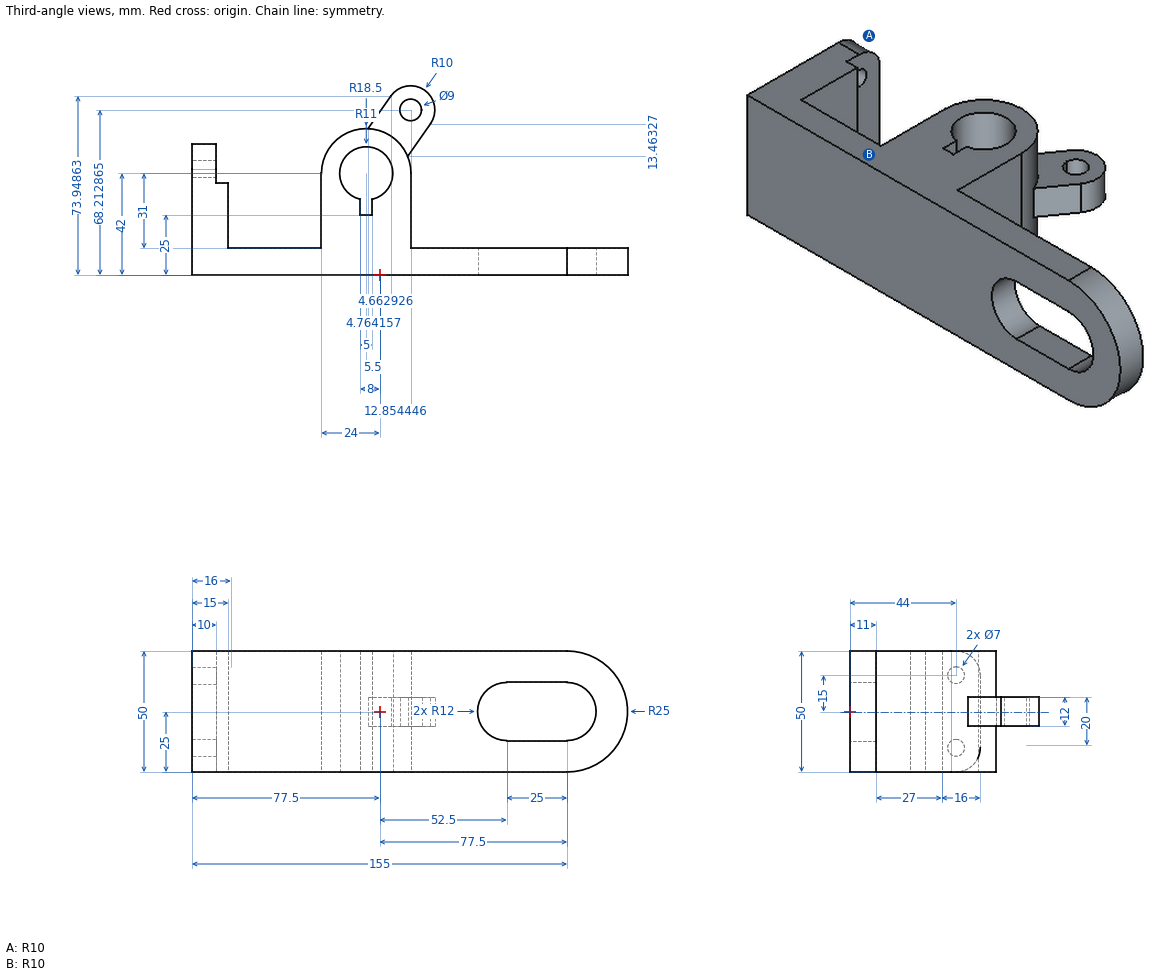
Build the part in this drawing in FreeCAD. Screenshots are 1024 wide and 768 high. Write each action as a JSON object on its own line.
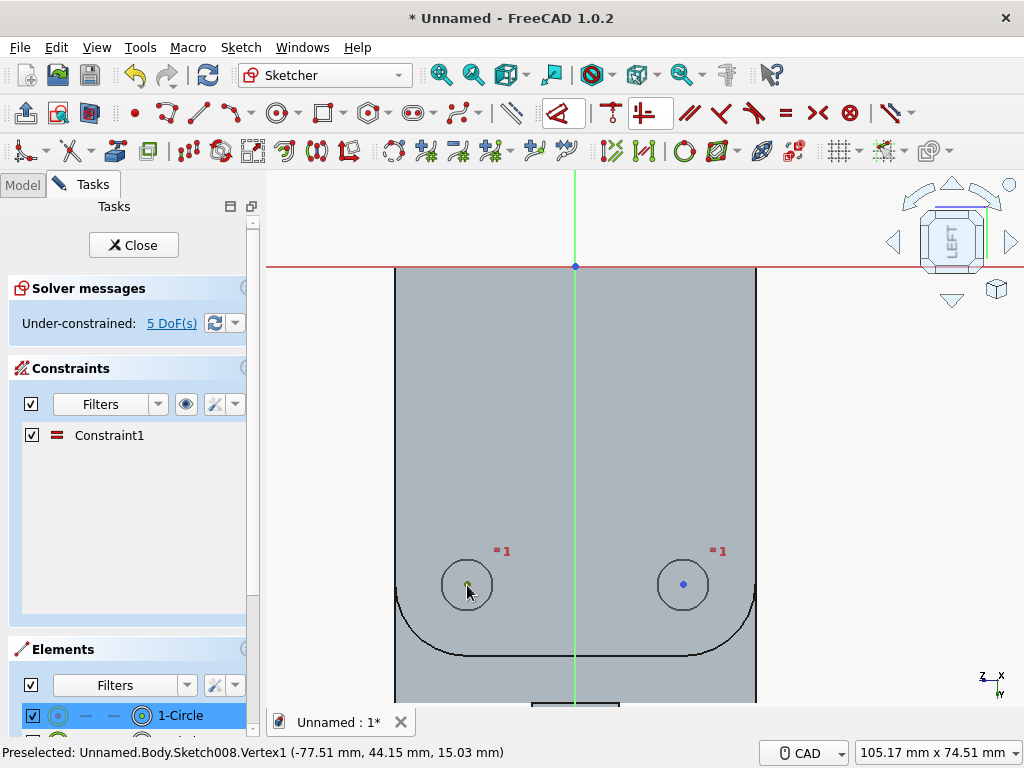
{"action": "left_click", "coordinate": [683, 585]}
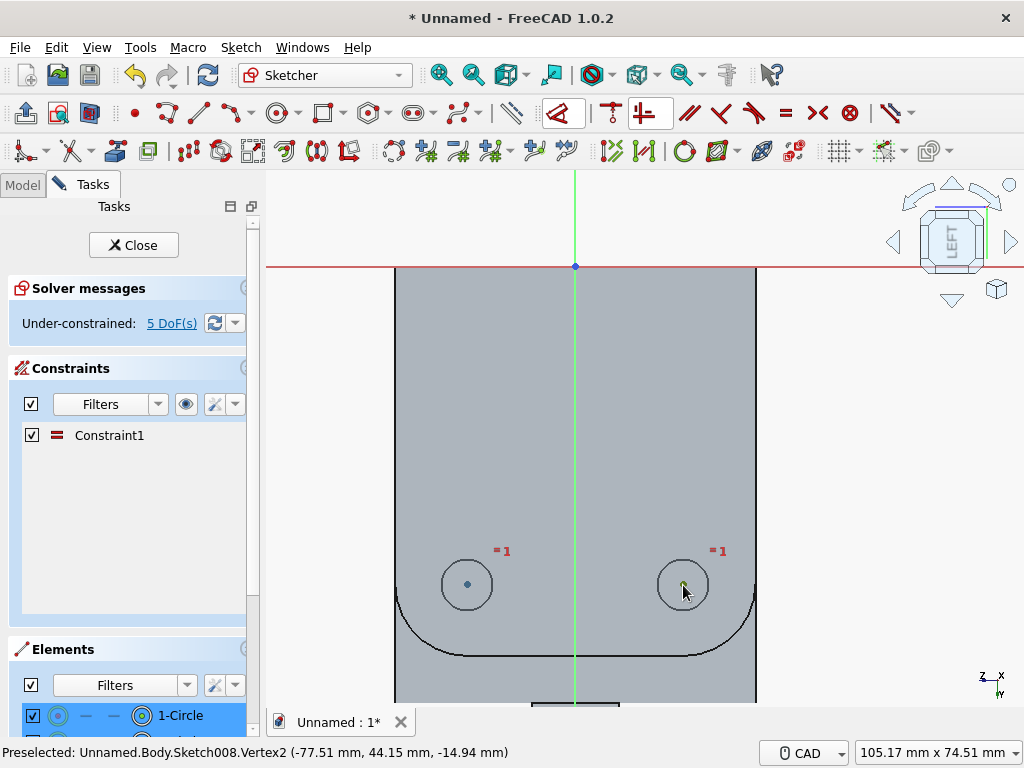
{"action": "left_click", "coordinate": [575, 645]}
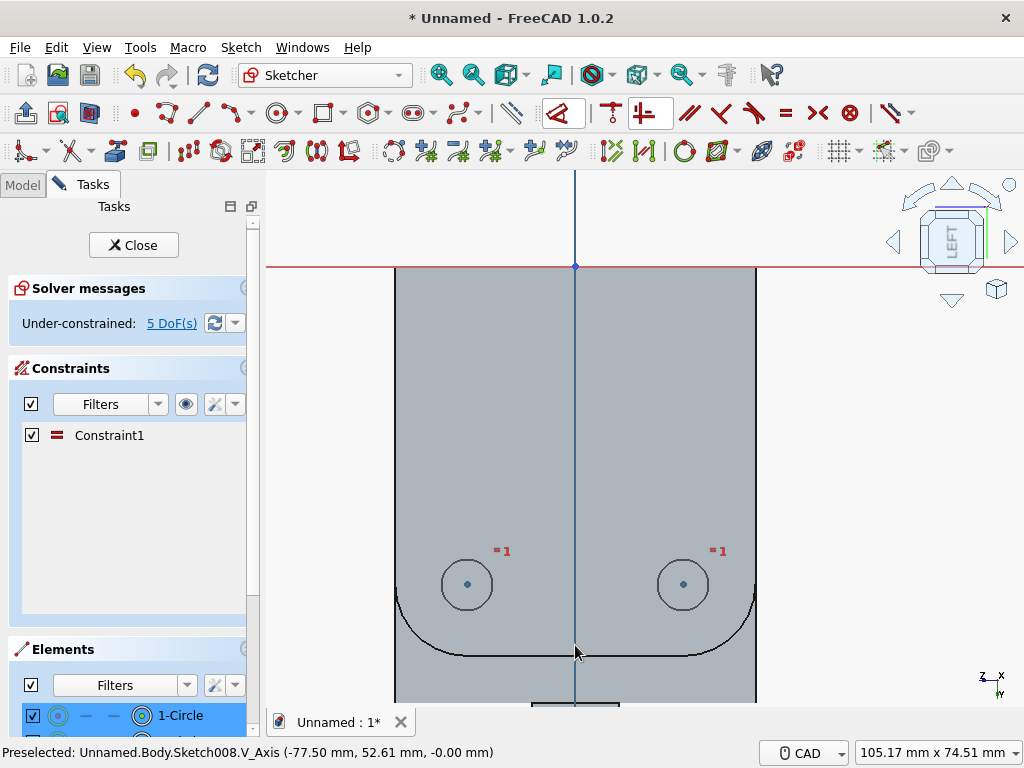
{"action": "left_click", "coordinate": [818, 114]}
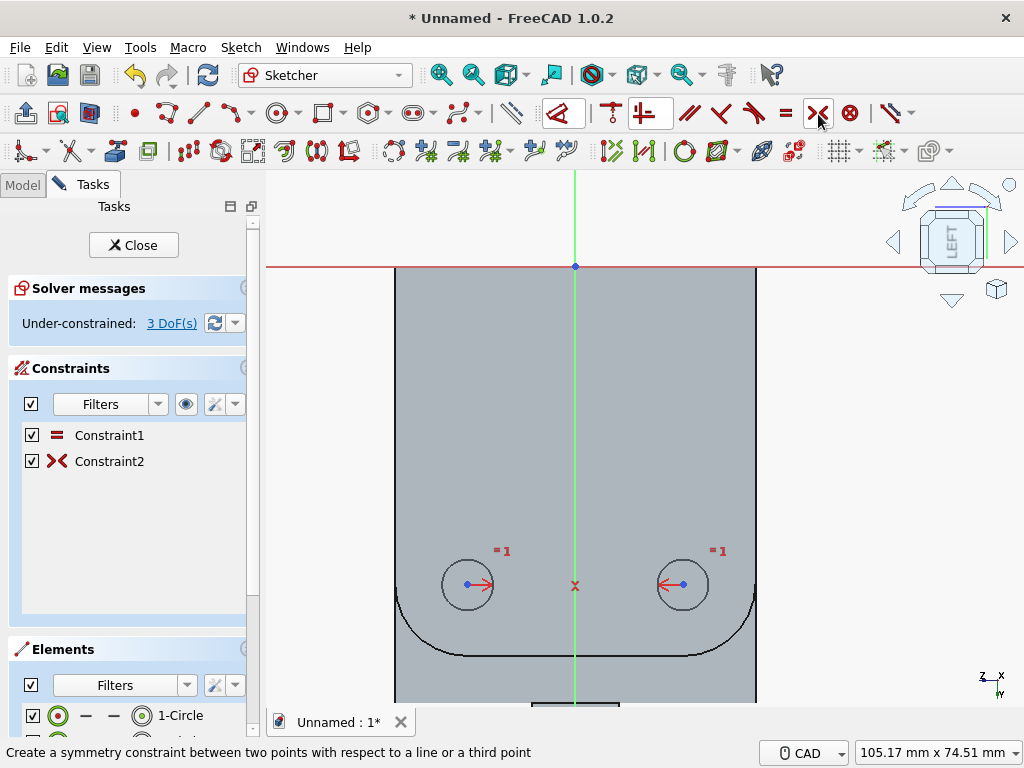
{"action": "left_click", "coordinate": [486, 567]}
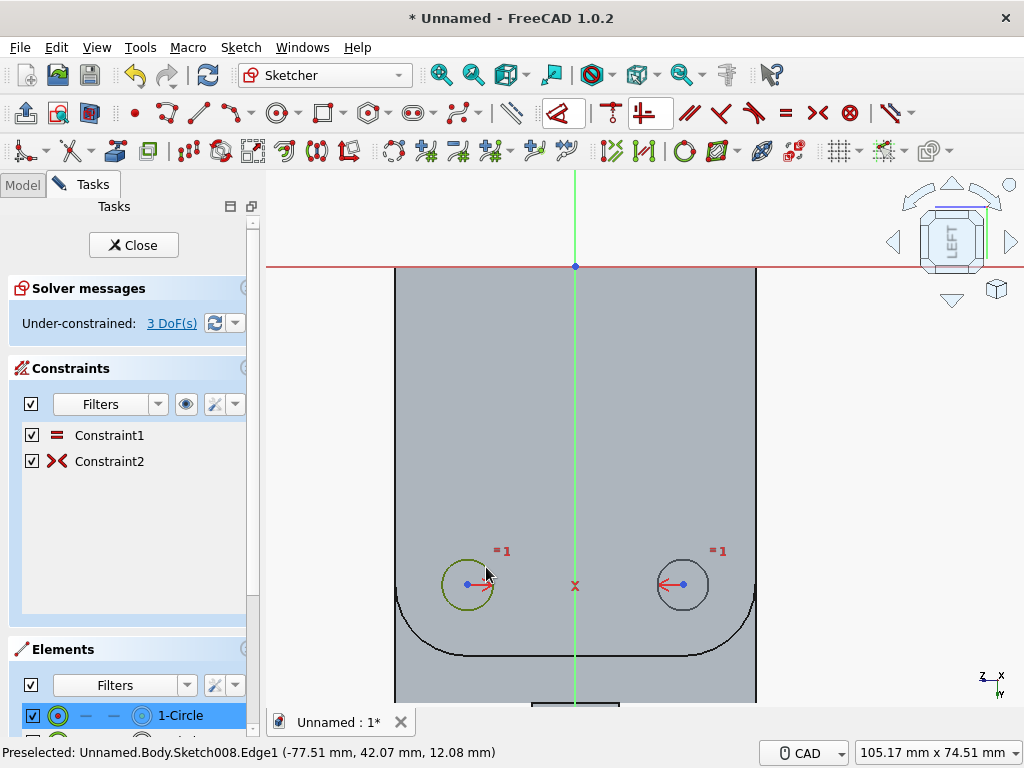
{"action": "key", "text": "k o"}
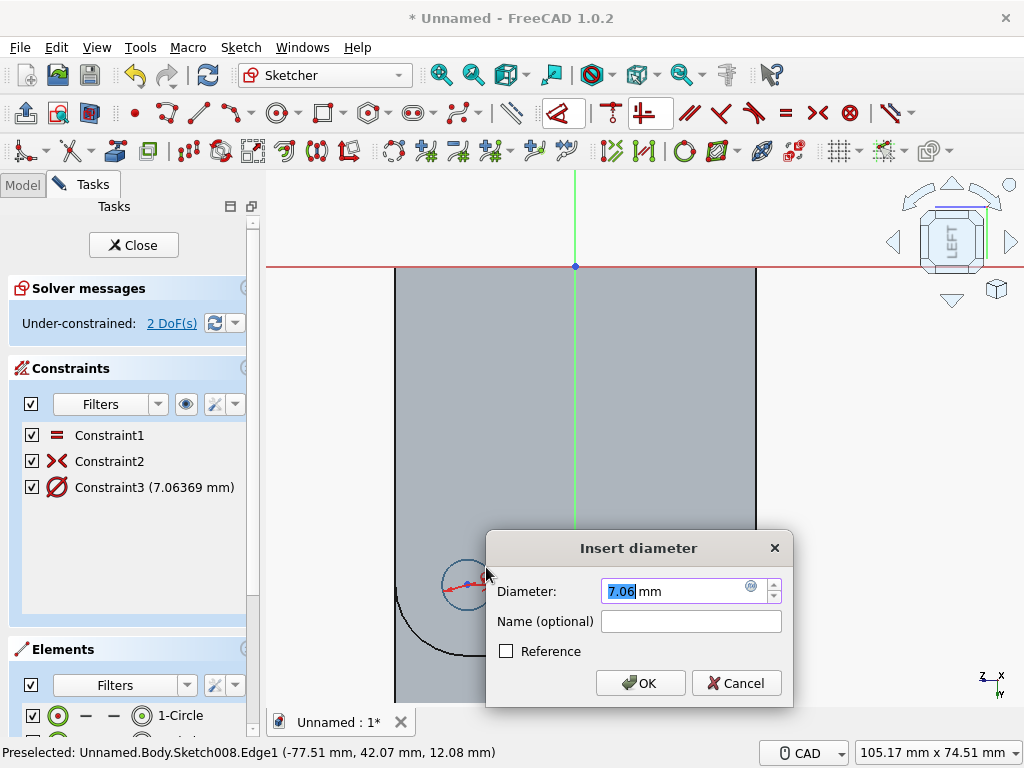
{"action": "type", "text": "7"}
{"action": "key", "text": "Return"}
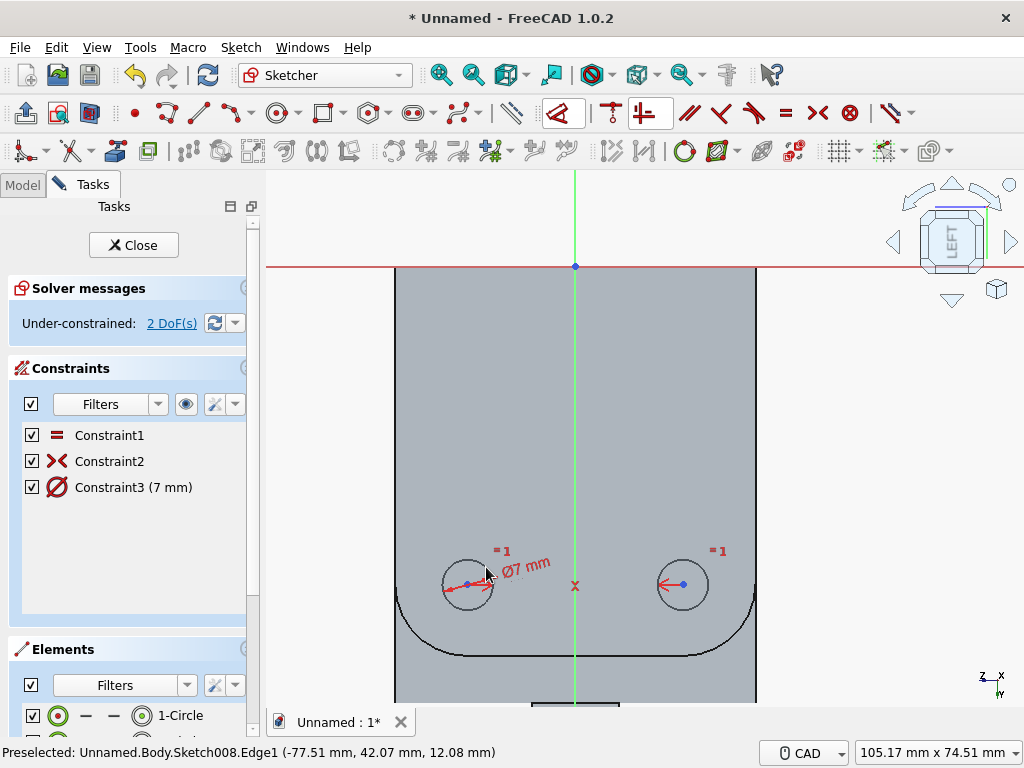
{"action": "left_click", "coordinate": [468, 585]}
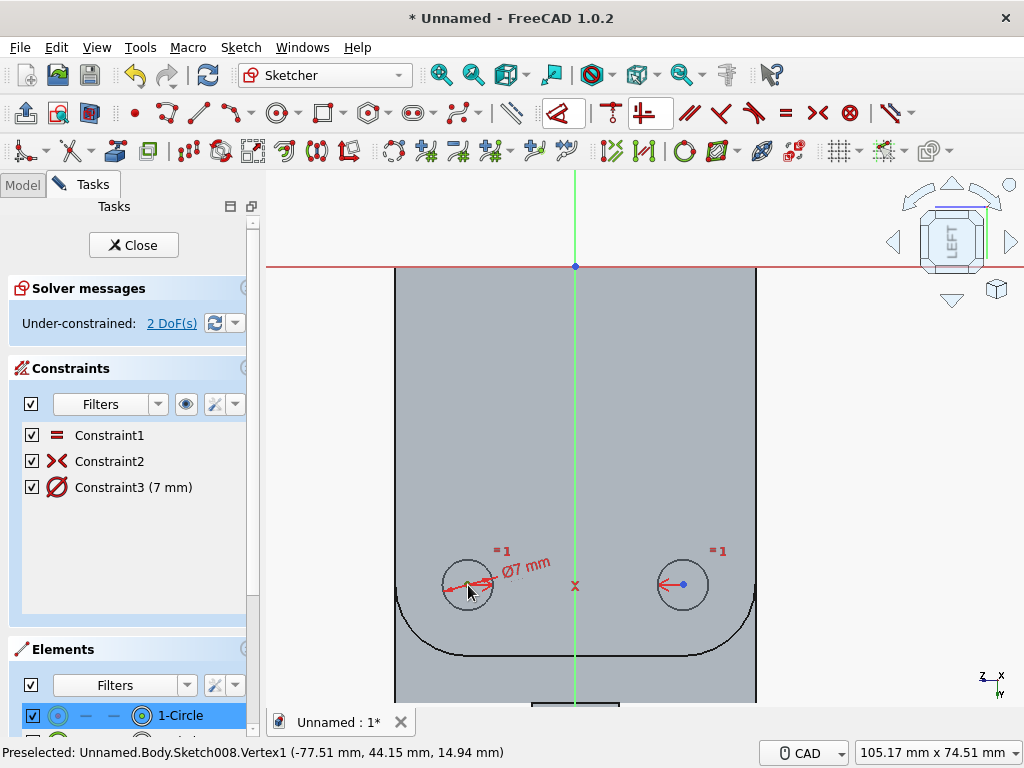
{"action": "left_click", "coordinate": [580, 114]}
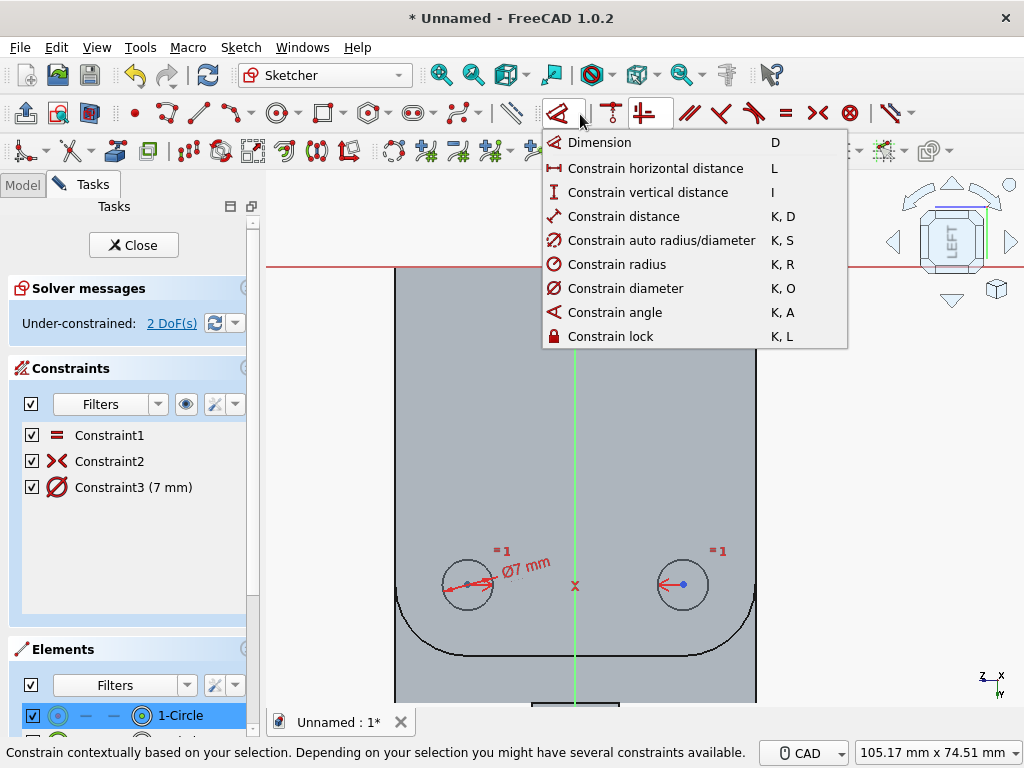
{"action": "left_click", "coordinate": [695, 168]}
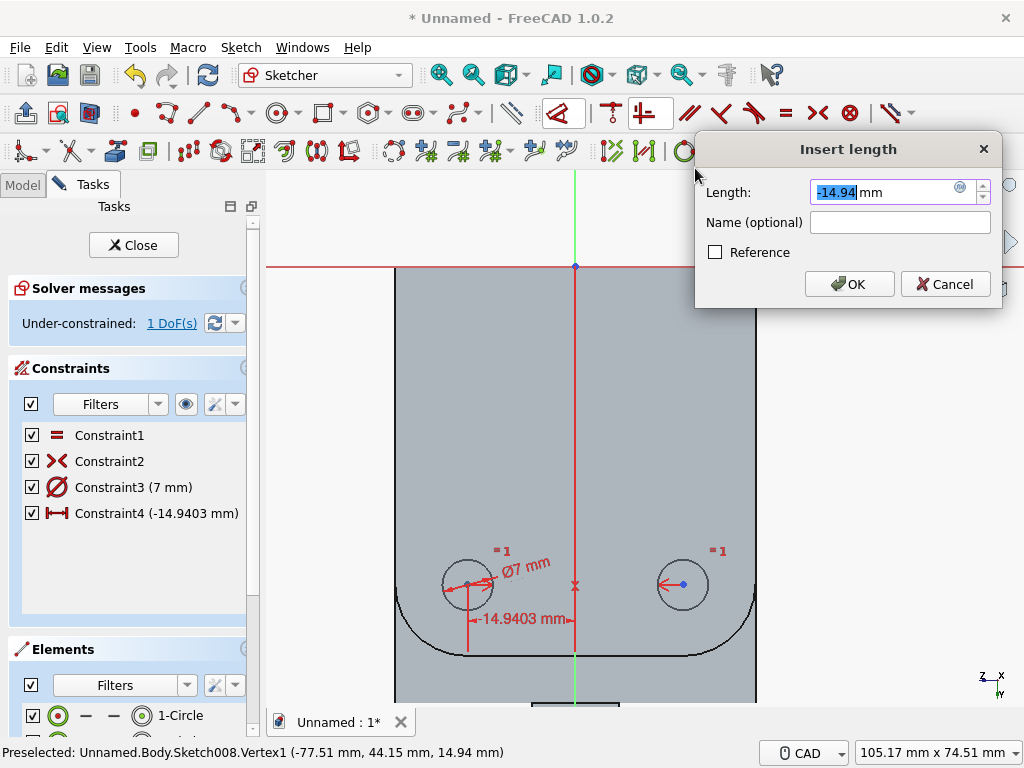
{"action": "type", "text": "-15"}
{"action": "key", "text": "Return"}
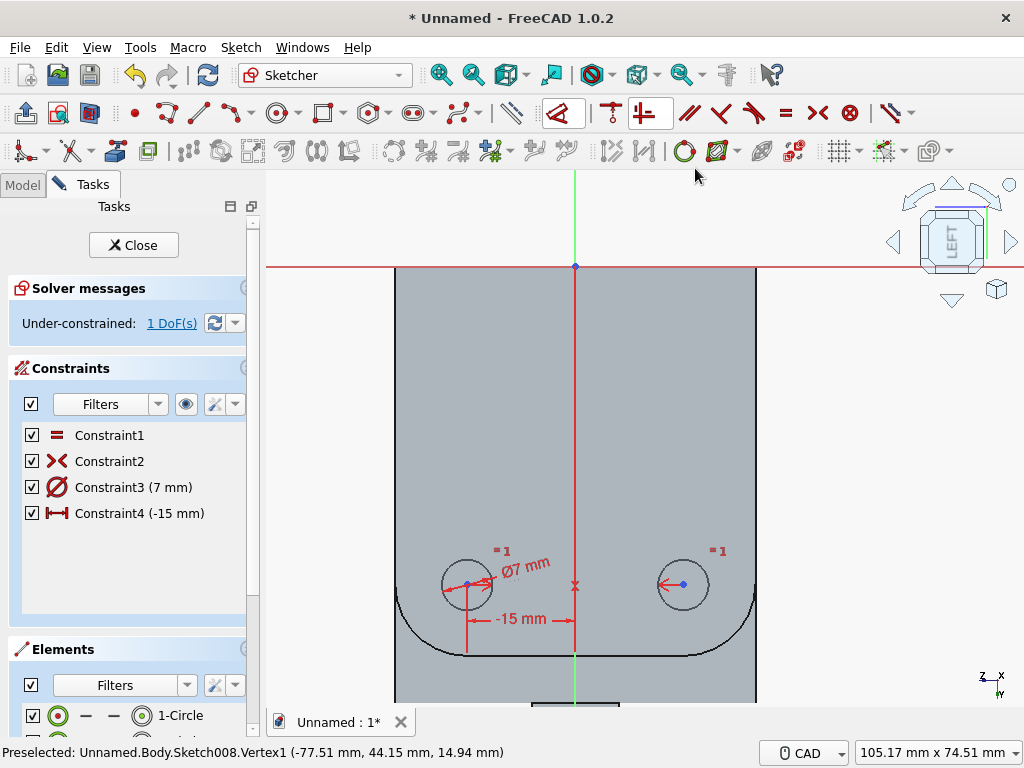
{"action": "left_click", "coordinate": [467, 585]}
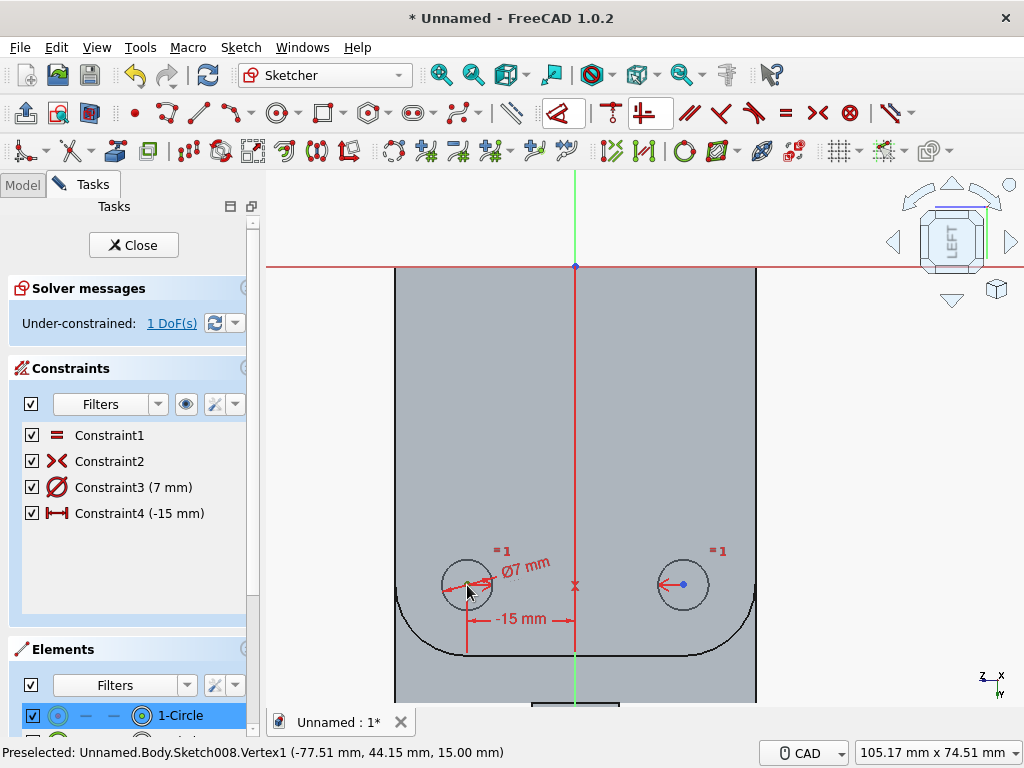
{"action": "key", "text": "i"}